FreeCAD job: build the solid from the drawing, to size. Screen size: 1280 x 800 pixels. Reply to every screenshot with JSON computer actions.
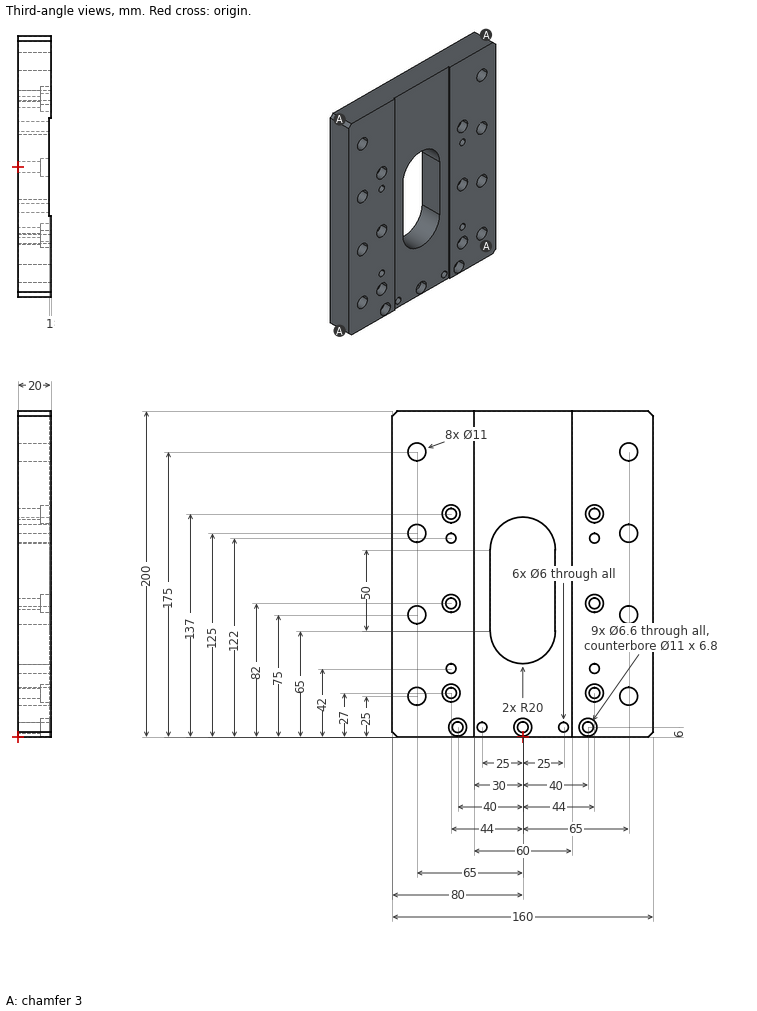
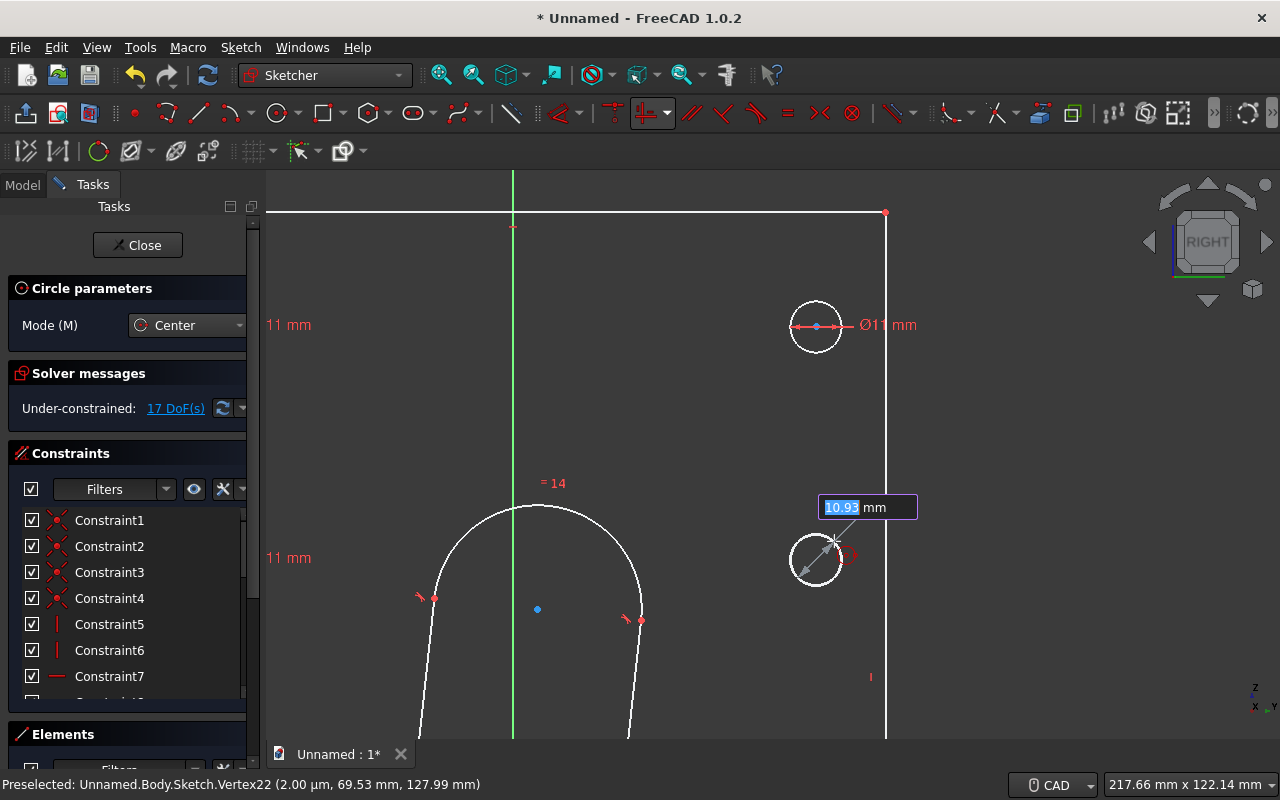
{"action": "type", "text": "11"}
{"action": "key", "text": "Return"}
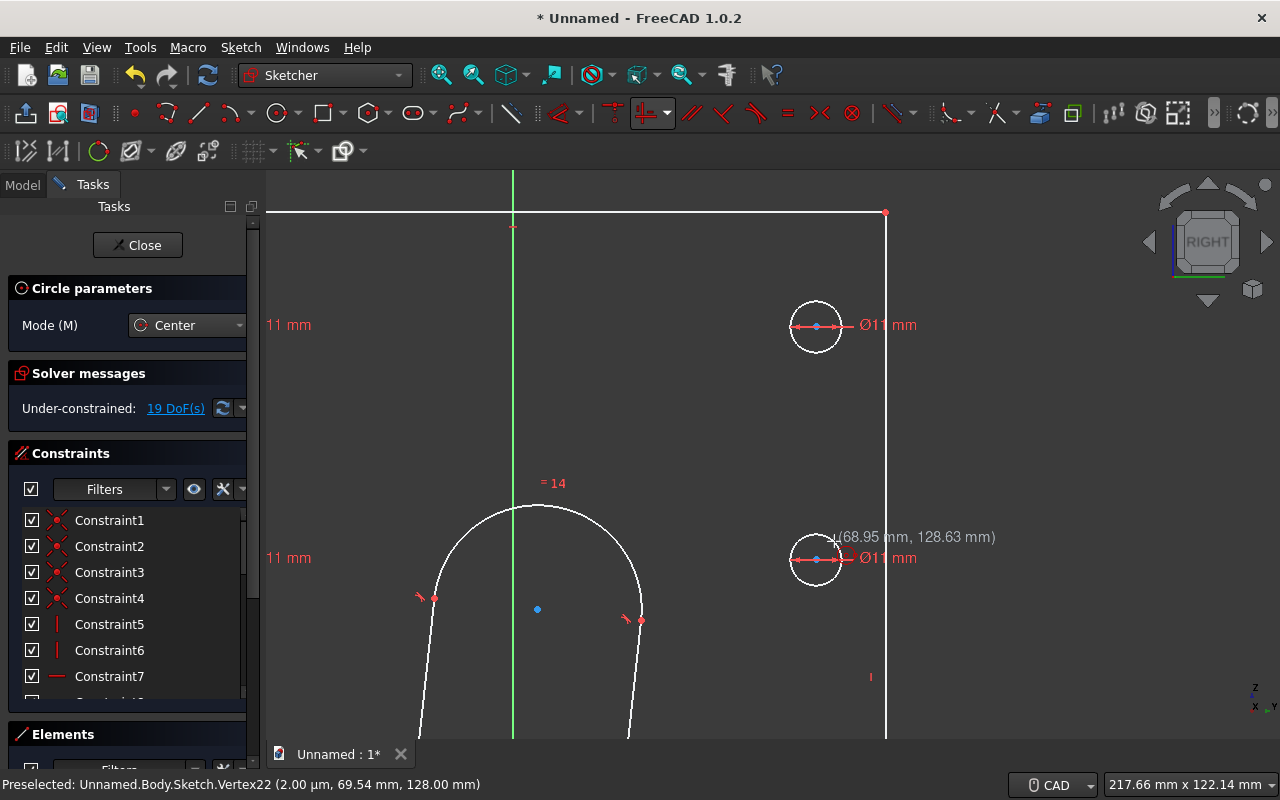
{"action": "scroll", "coordinate": [816, 326], "scroll_direction": "down", "scroll_amount": 5}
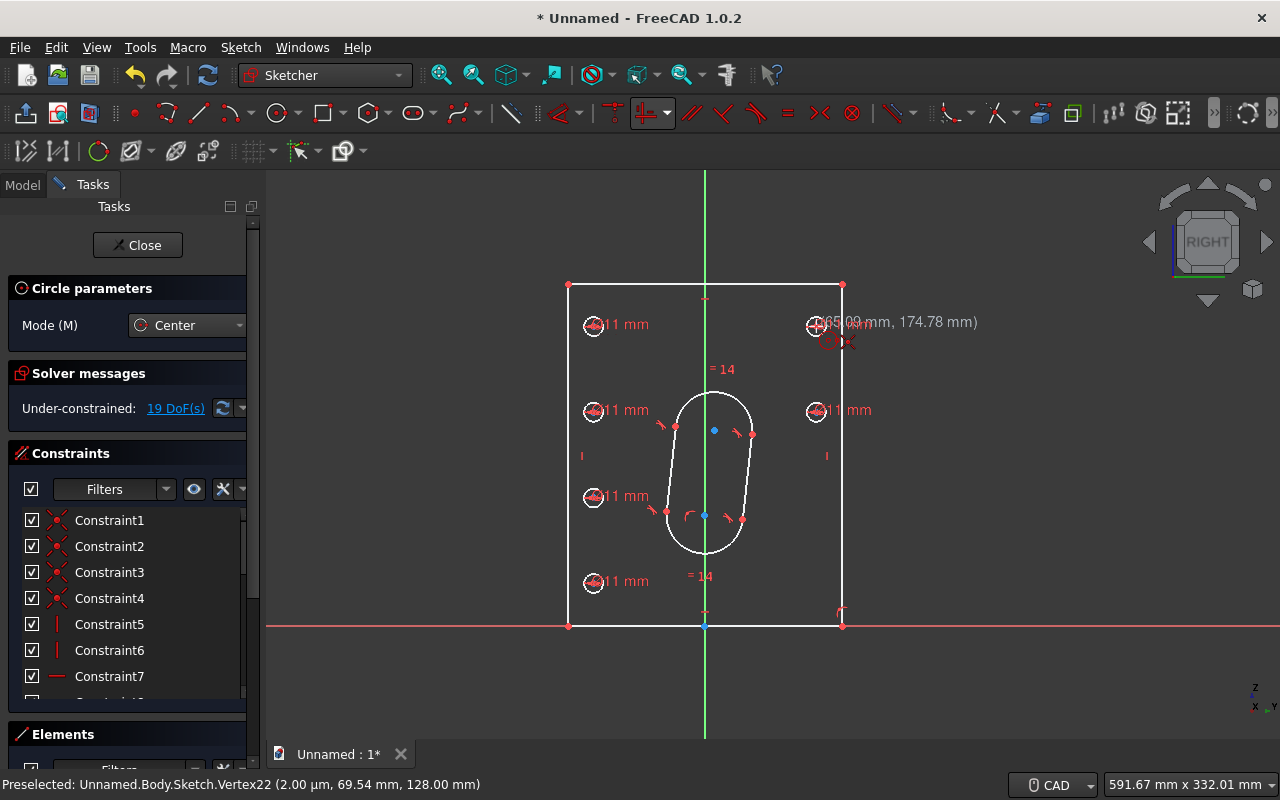
{"action": "scroll", "coordinate": [816, 498], "scroll_direction": "up", "scroll_amount": 5}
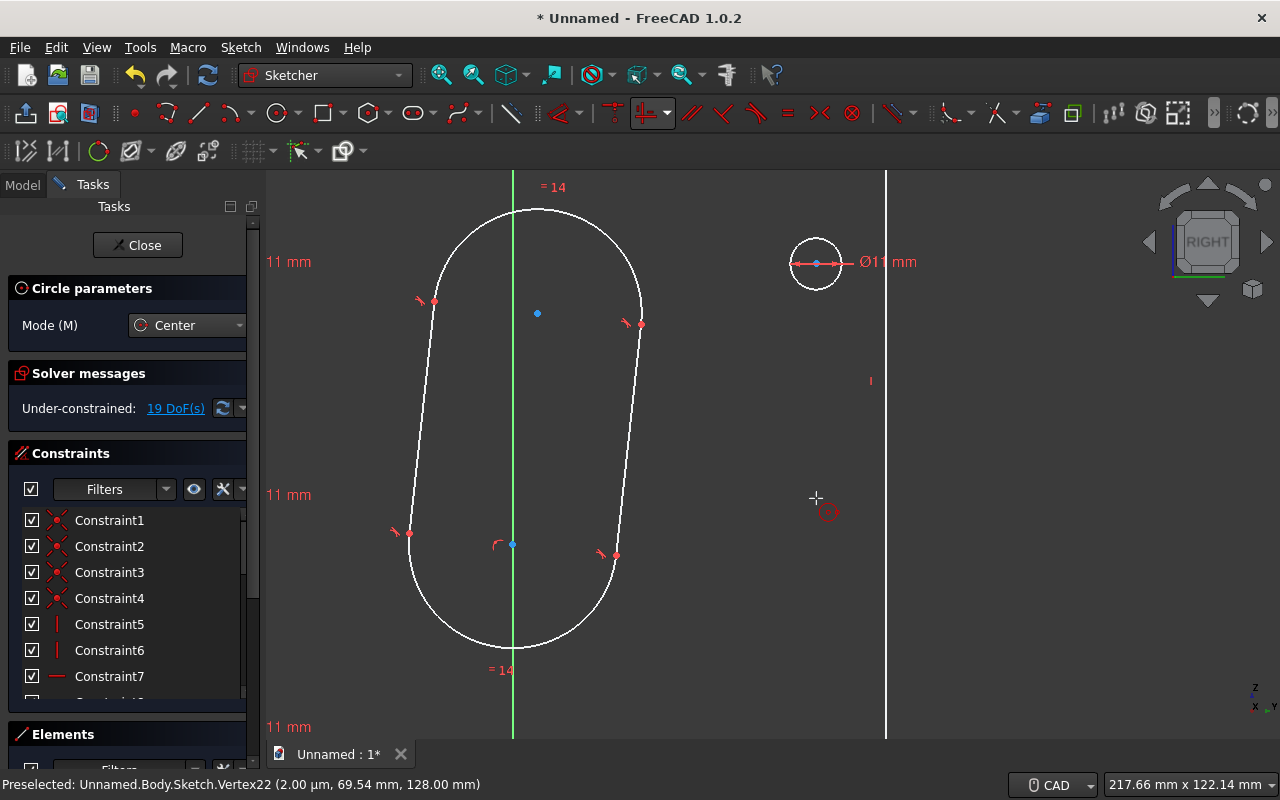
{"action": "left_click", "coordinate": [816, 496]}
{"action": "mouse_move", "coordinate": [834, 478]}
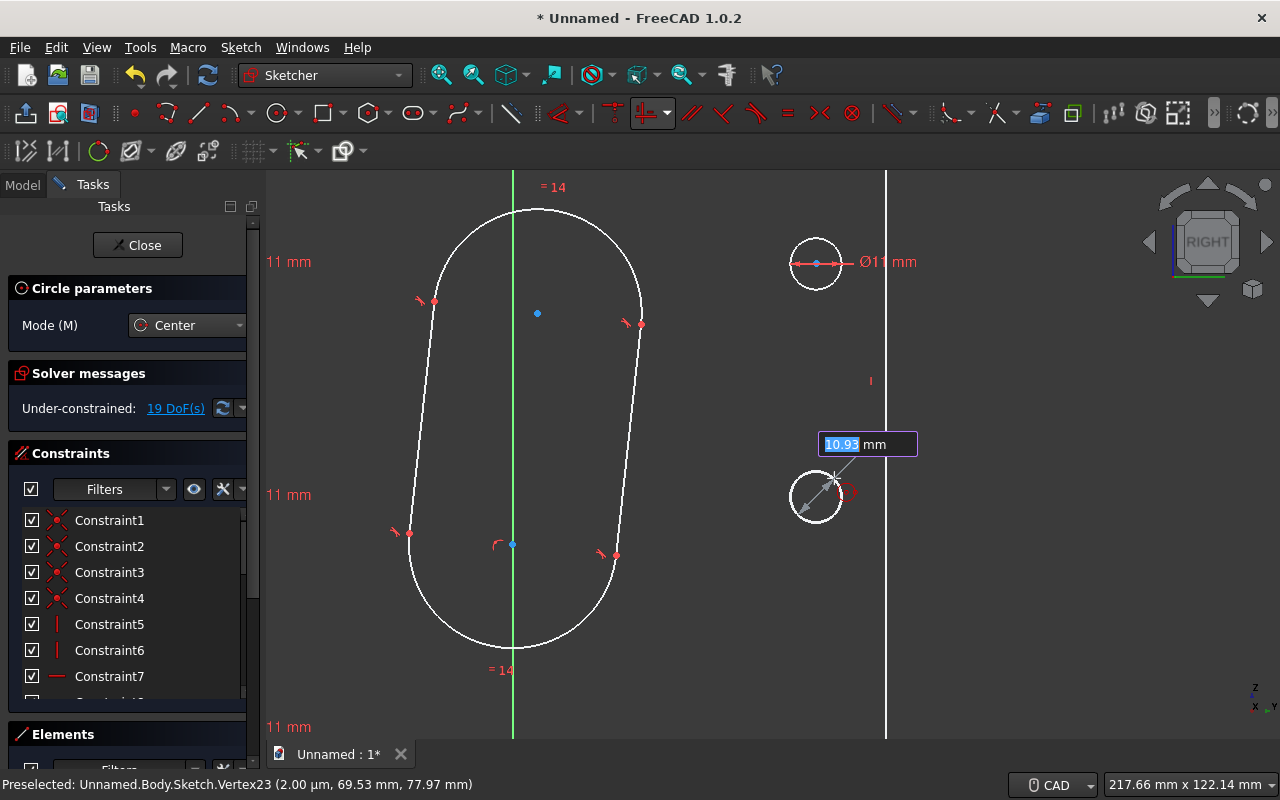
{"action": "type", "text": "11"}
{"action": "key", "text": "Return"}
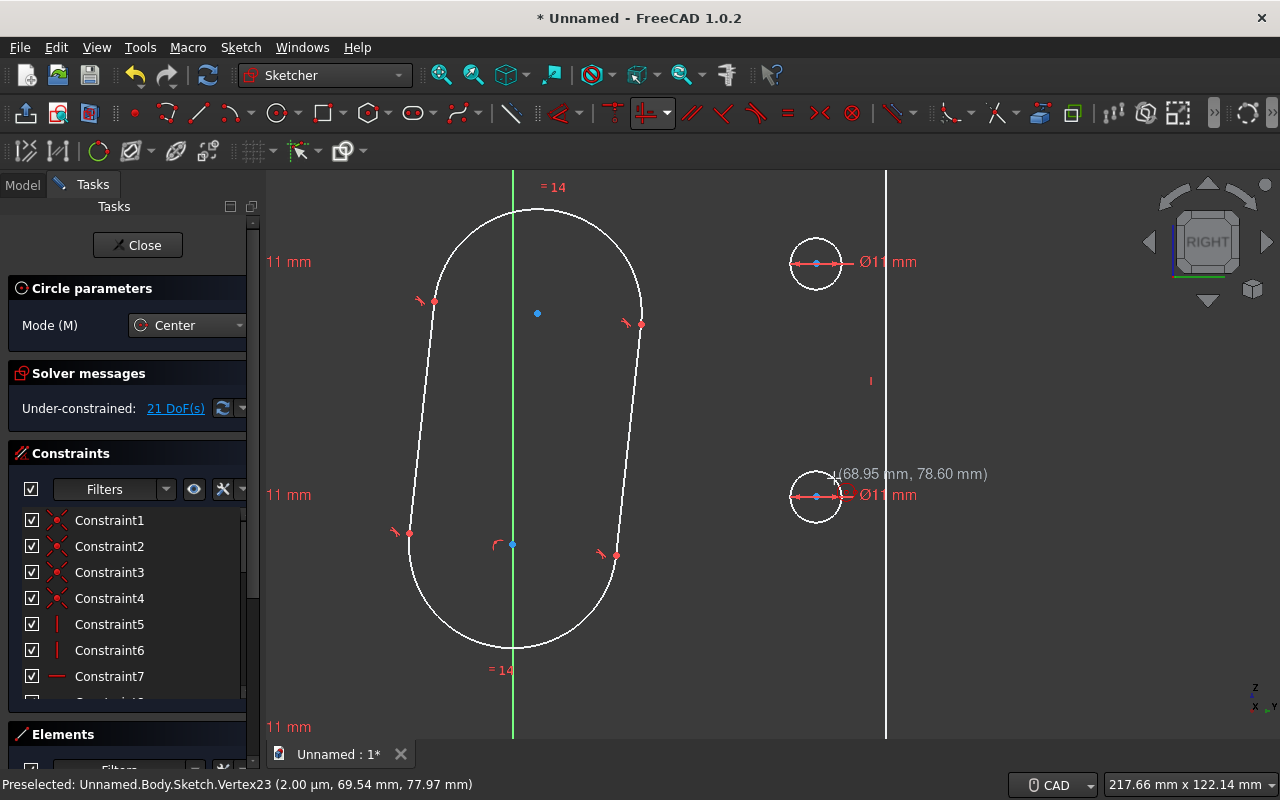
{"action": "scroll", "coordinate": [816, 498], "scroll_direction": "down", "scroll_amount": 5}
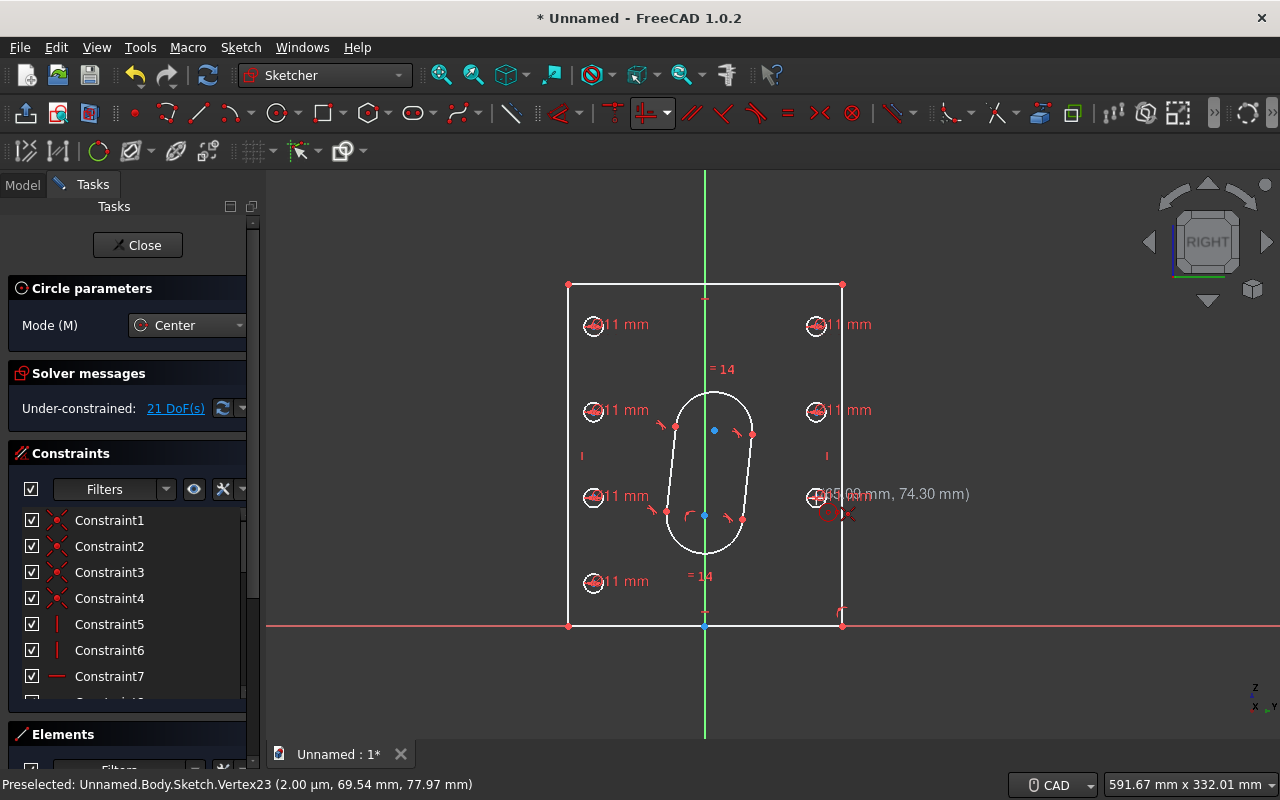
{"action": "scroll", "coordinate": [816, 583], "scroll_direction": "up", "scroll_amount": 5}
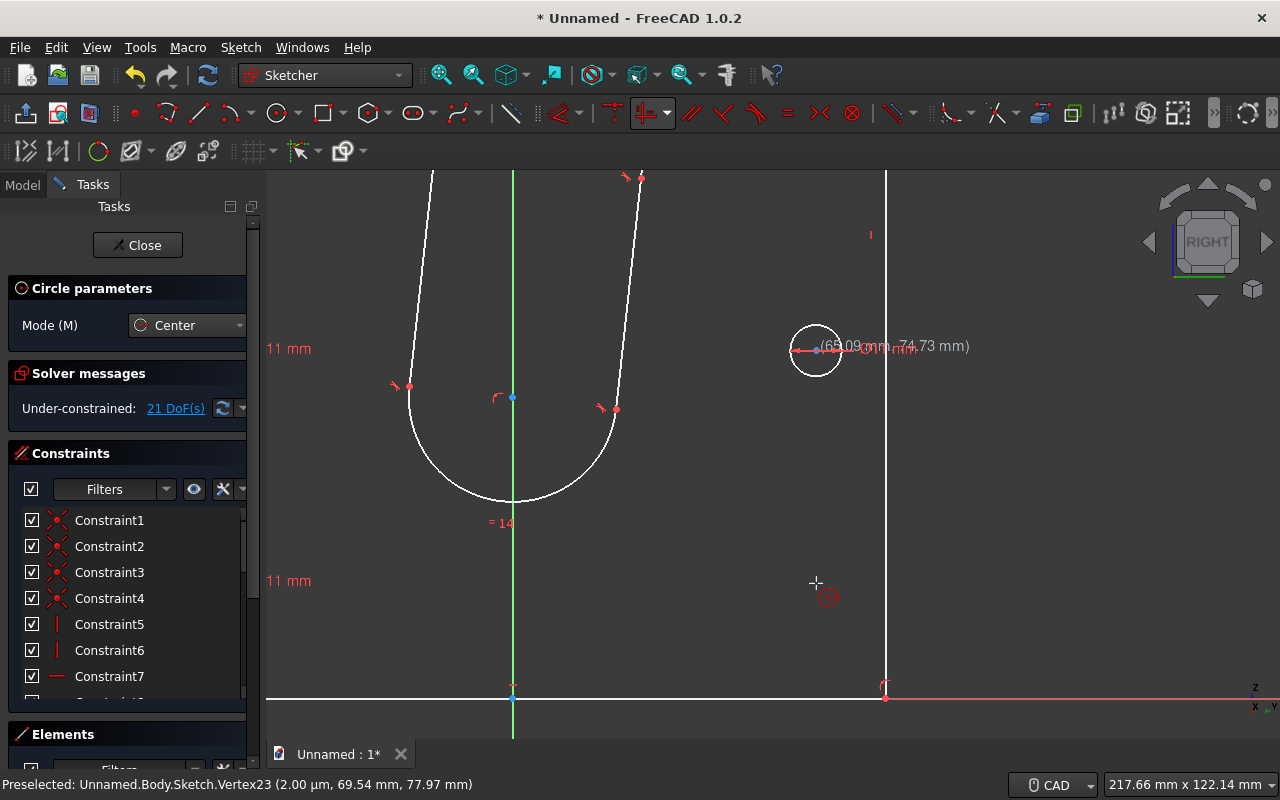
{"action": "left_click", "coordinate": [816, 582]}
{"action": "mouse_move", "coordinate": [834, 564]}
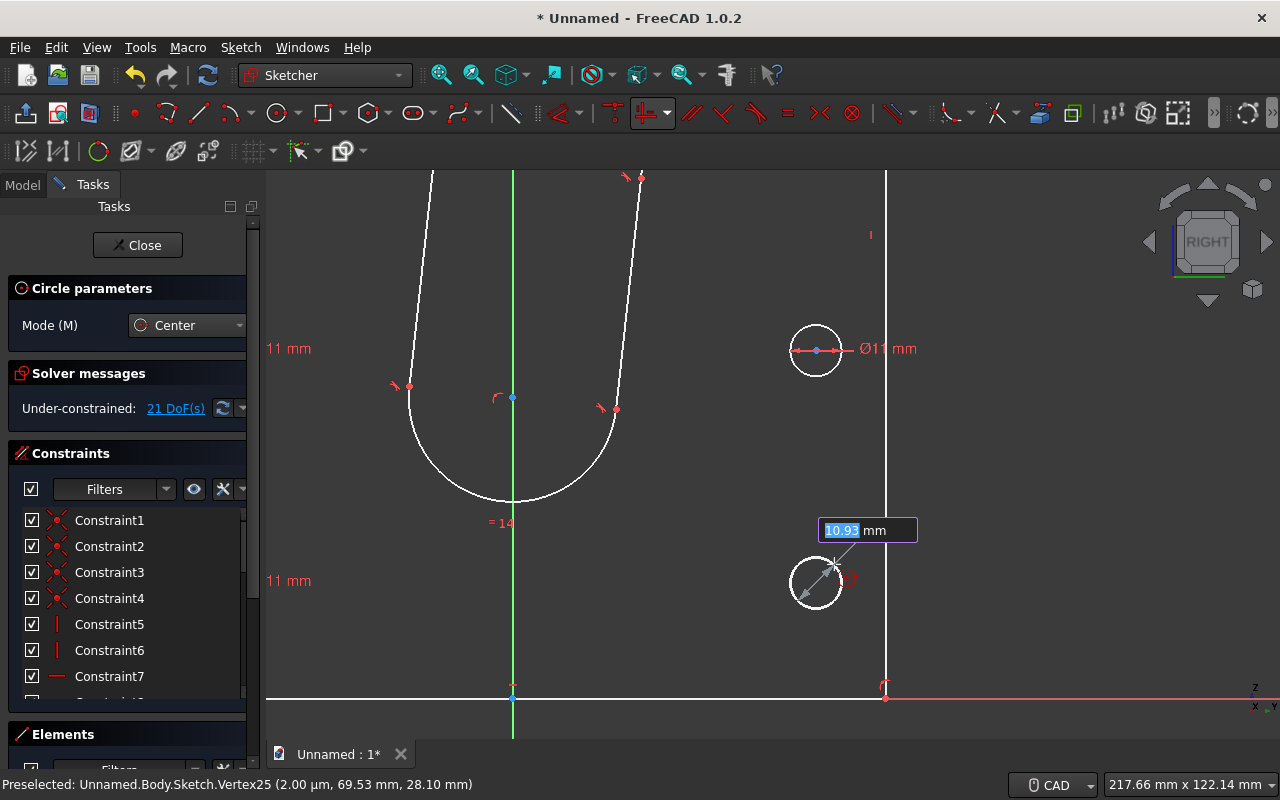
{"action": "type", "text": "11"}
{"action": "key", "text": "Return"}
{"action": "key", "text": "Escape"}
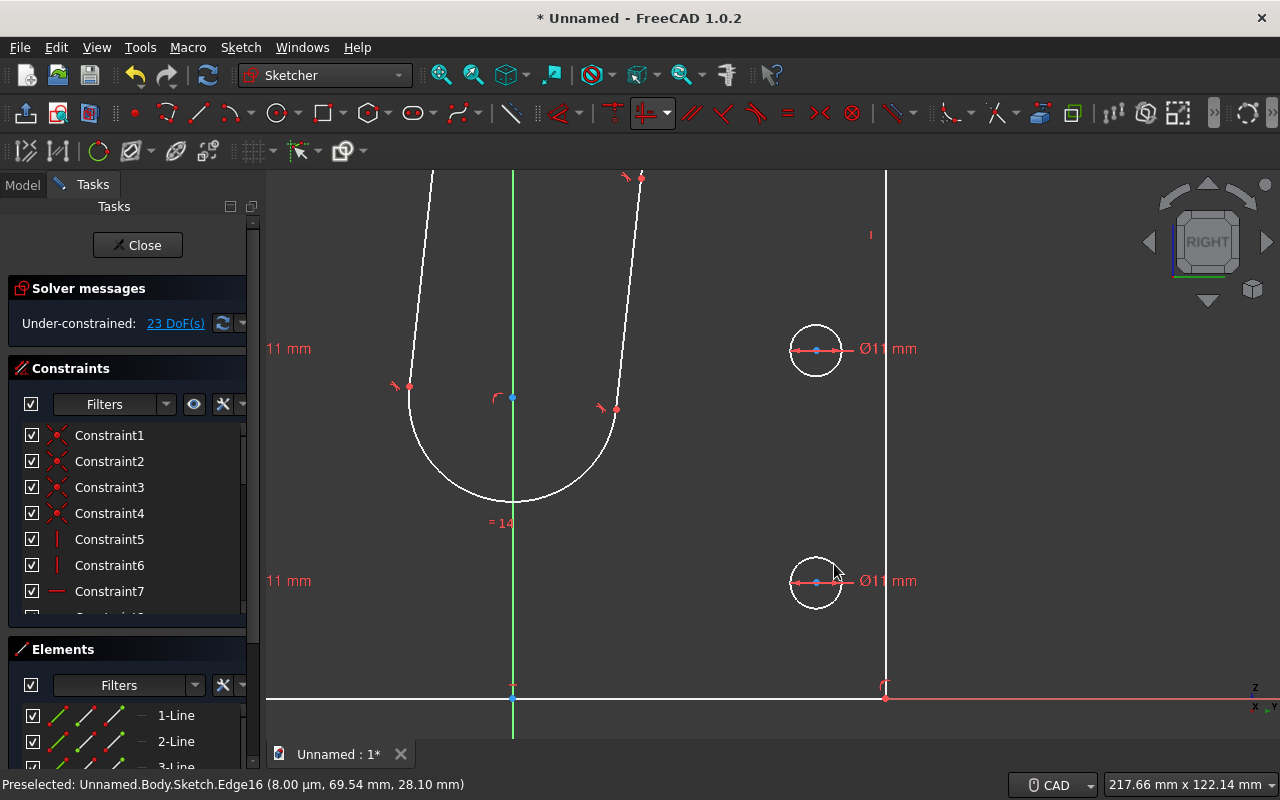
{"action": "left_click", "coordinate": [417, 317]}